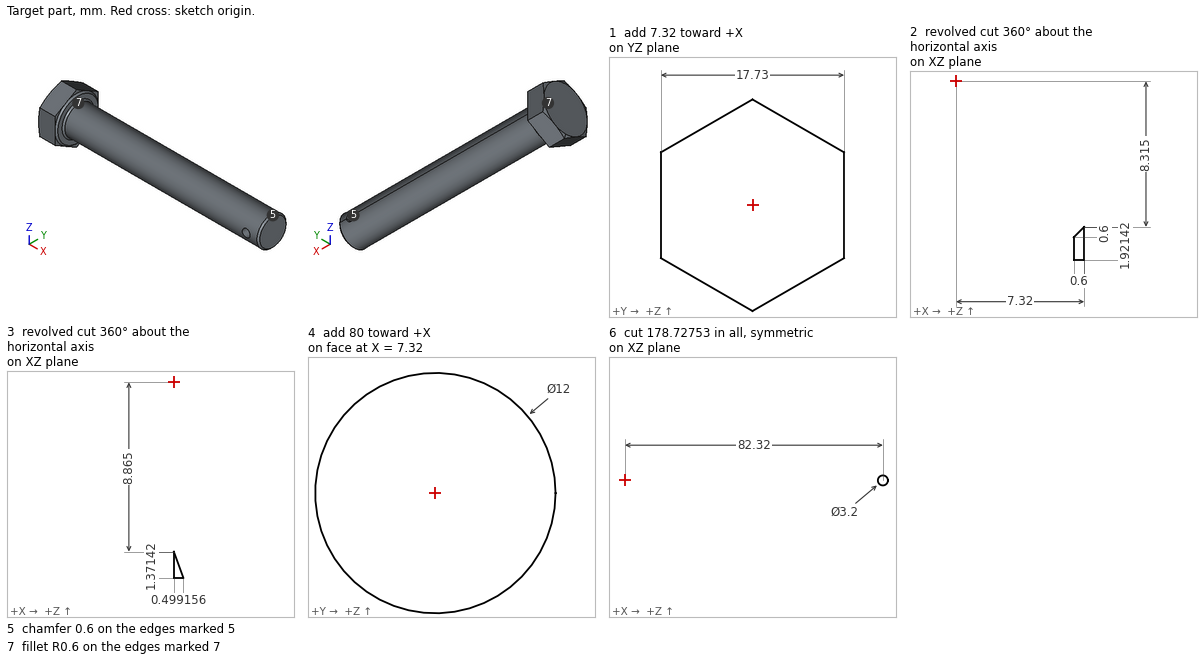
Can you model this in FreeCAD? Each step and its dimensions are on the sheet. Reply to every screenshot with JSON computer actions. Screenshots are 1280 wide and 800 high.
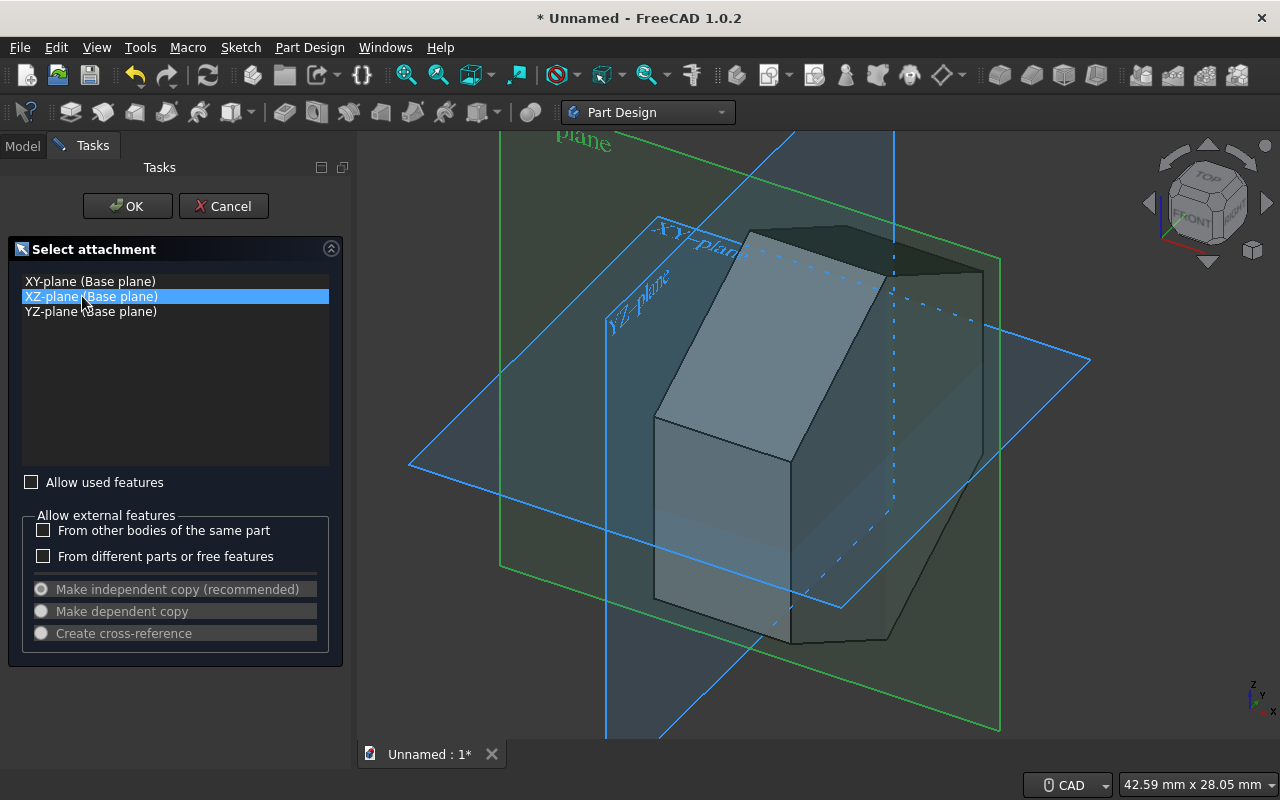
{"action": "left_click", "coordinate": [128, 206]}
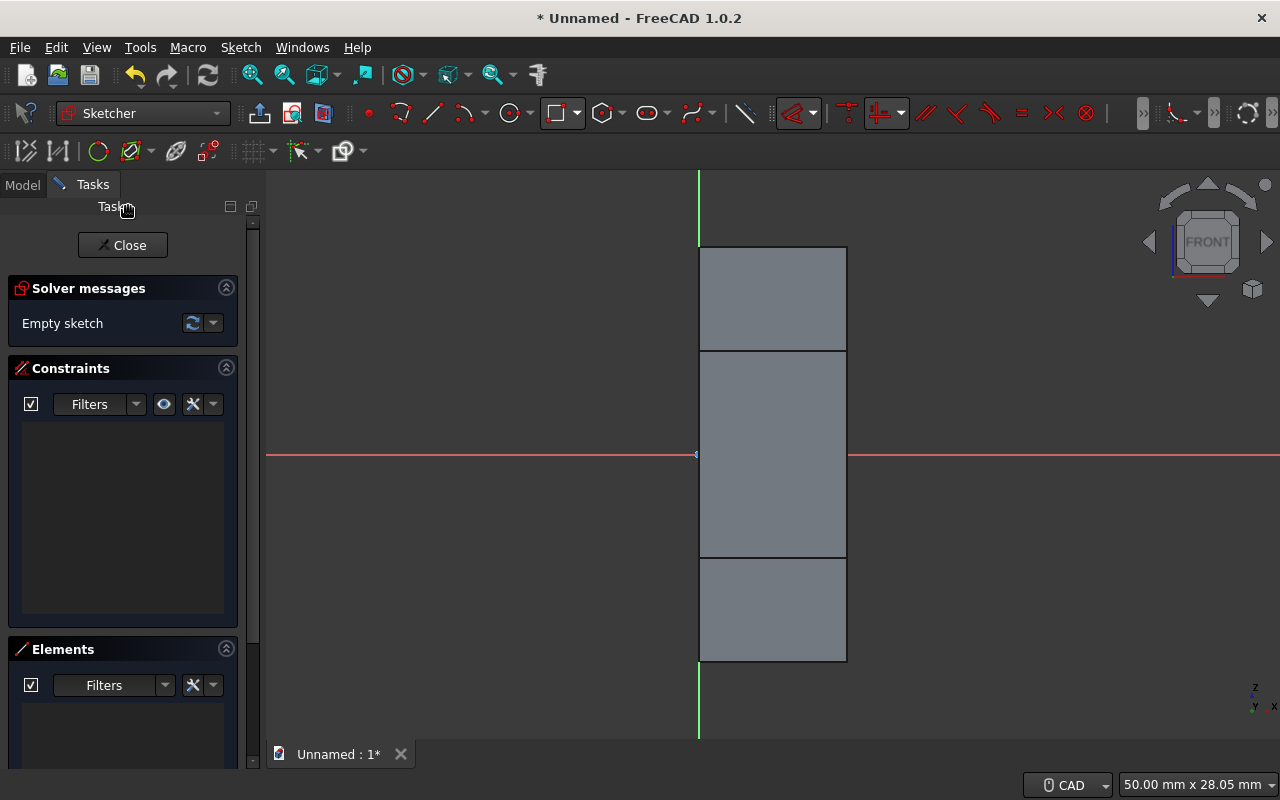
{"action": "left_click", "coordinate": [324, 114]}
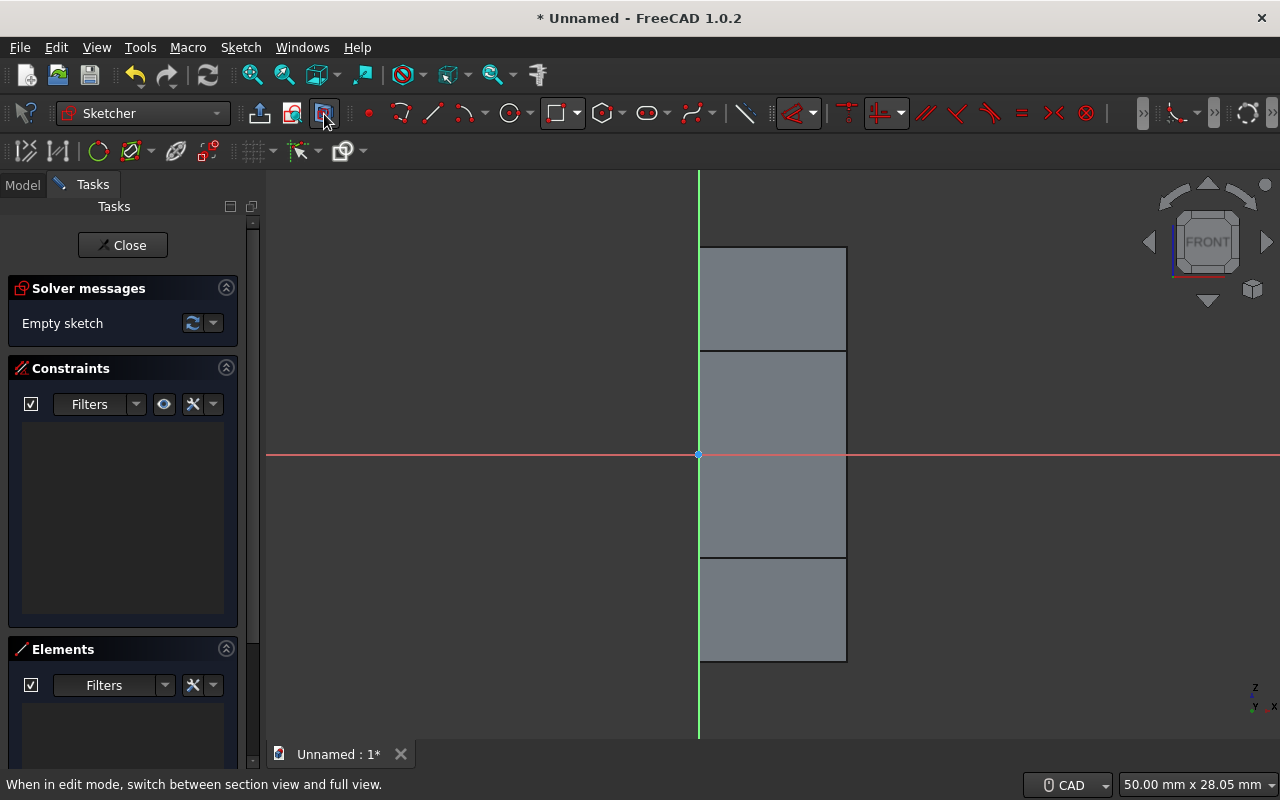
{"action": "scroll", "coordinate": [858, 666], "scroll_direction": "up", "scroll_amount": 11}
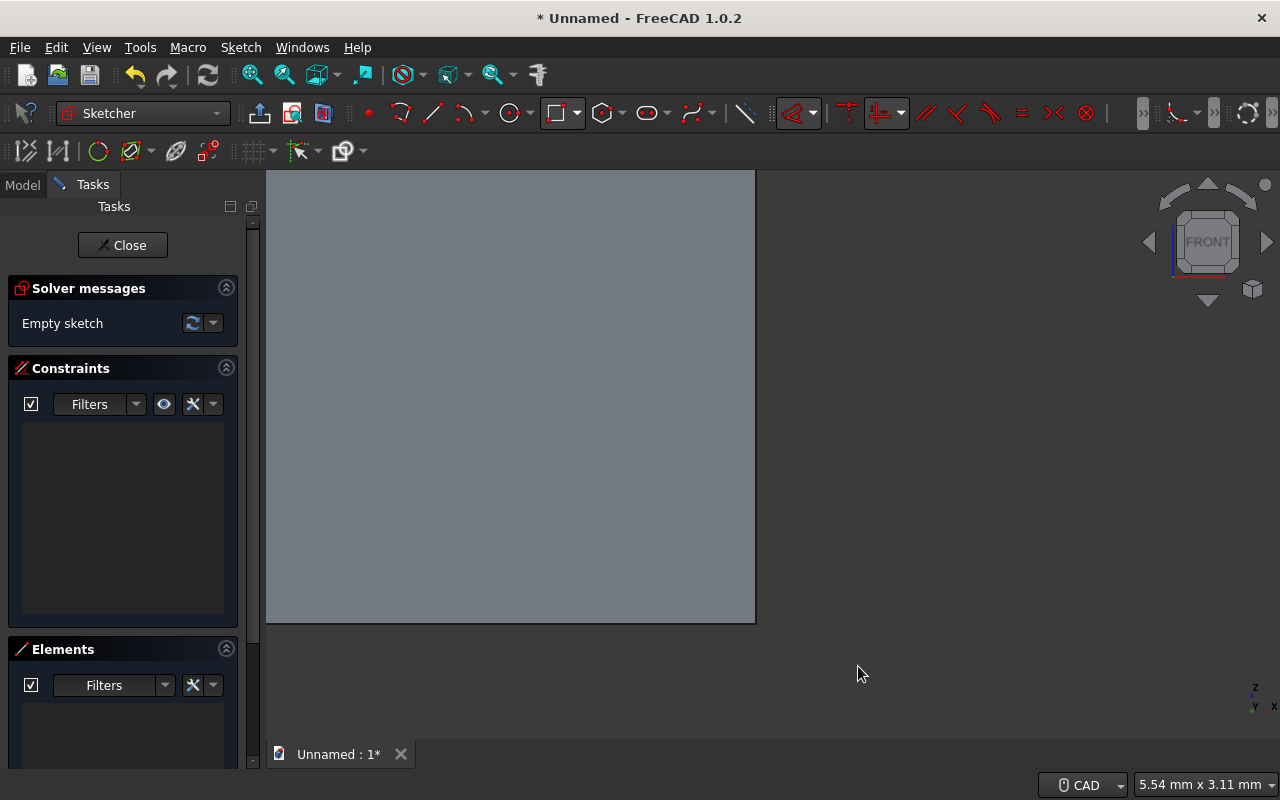
{"action": "left_click", "coordinate": [402, 114]}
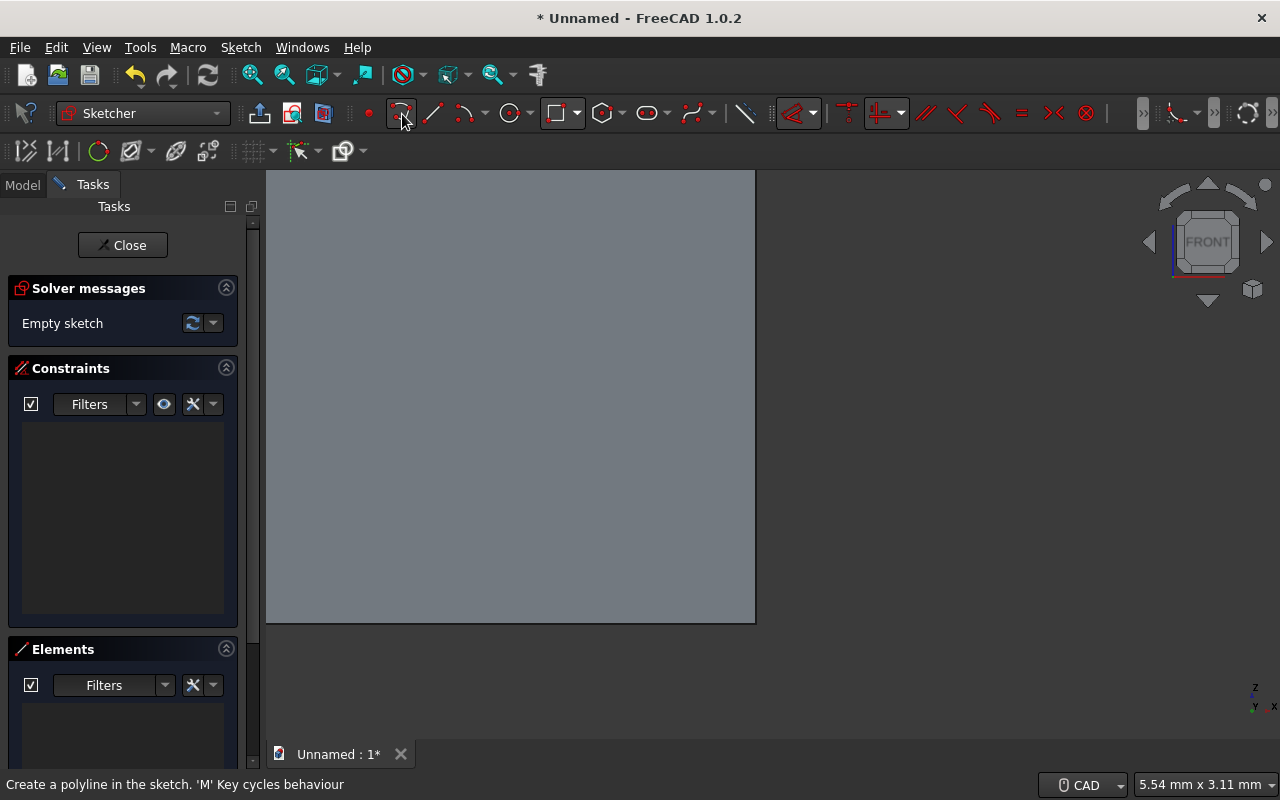
{"action": "left_click", "coordinate": [756, 272]}
{"action": "left_click", "coordinate": [756, 624]}
{"action": "left_click", "coordinate": [646, 624]}
{"action": "left_click", "coordinate": [646, 382]}
{"action": "left_click", "coordinate": [756, 273]}
{"action": "key", "text": "Escape"}
{"action": "key", "text": "Escape"}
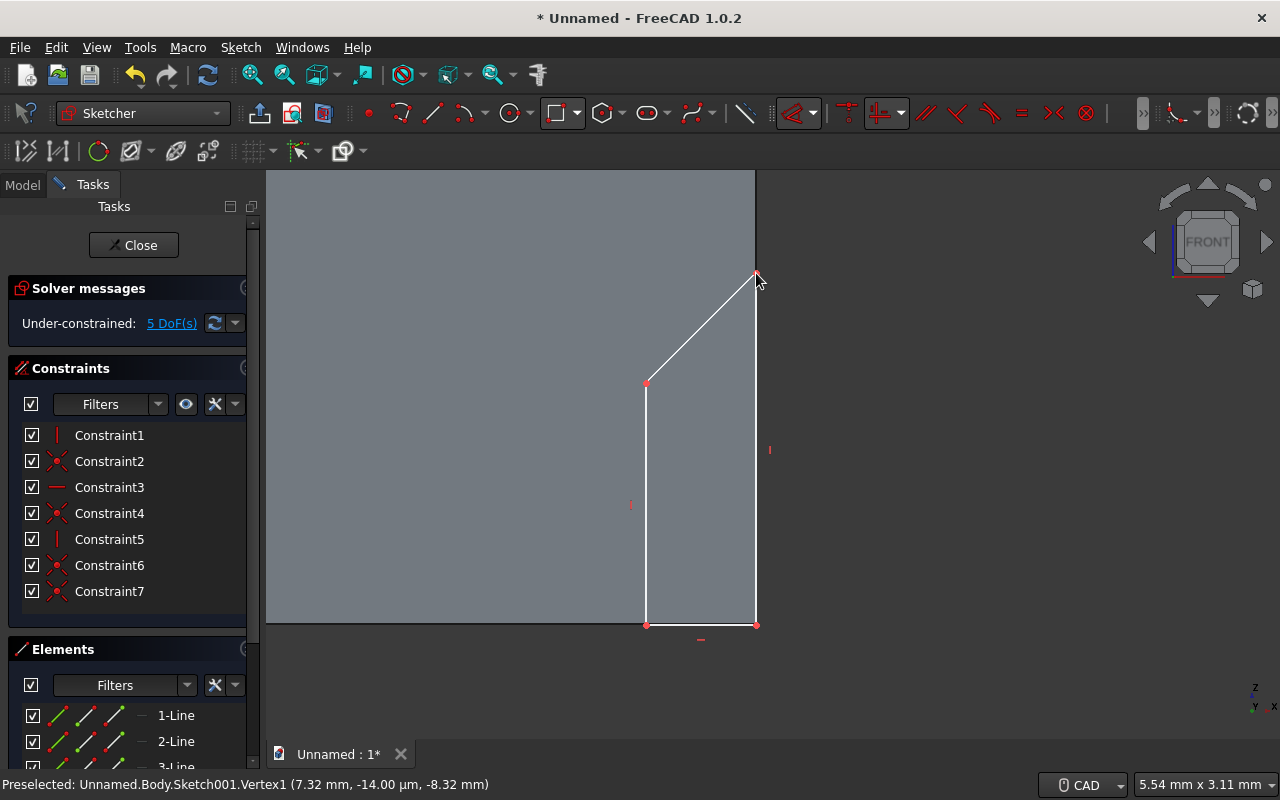
{"action": "left_click", "coordinate": [723, 625]}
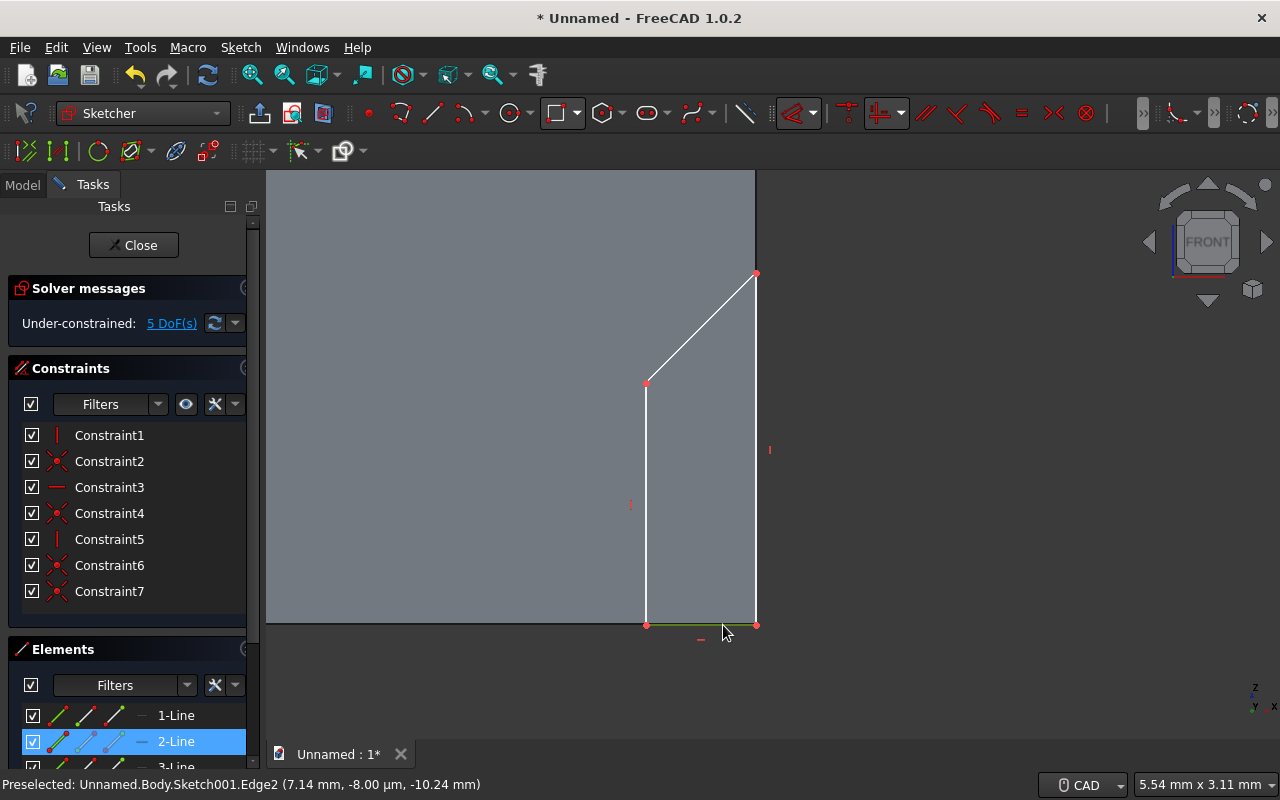
{"action": "left_click", "coordinate": [816, 114]}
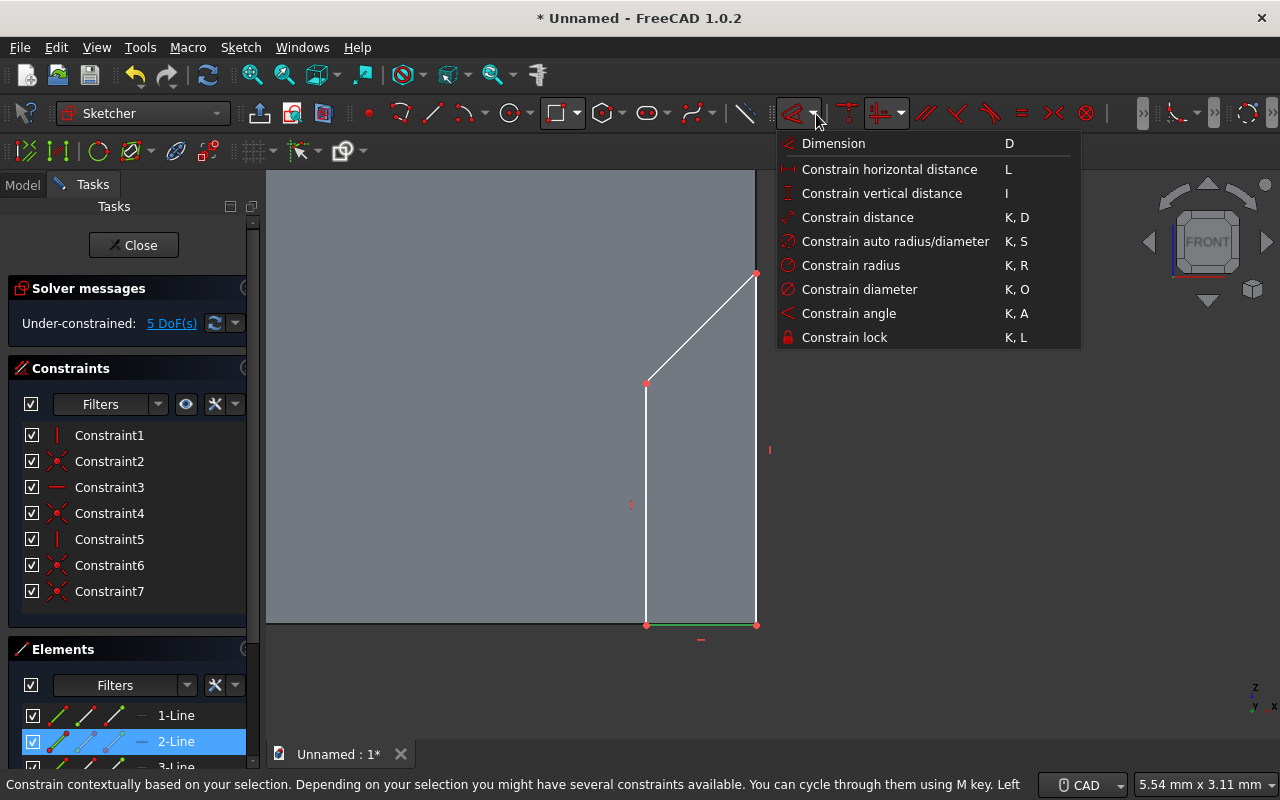
{"action": "left_click", "coordinate": [929, 169]}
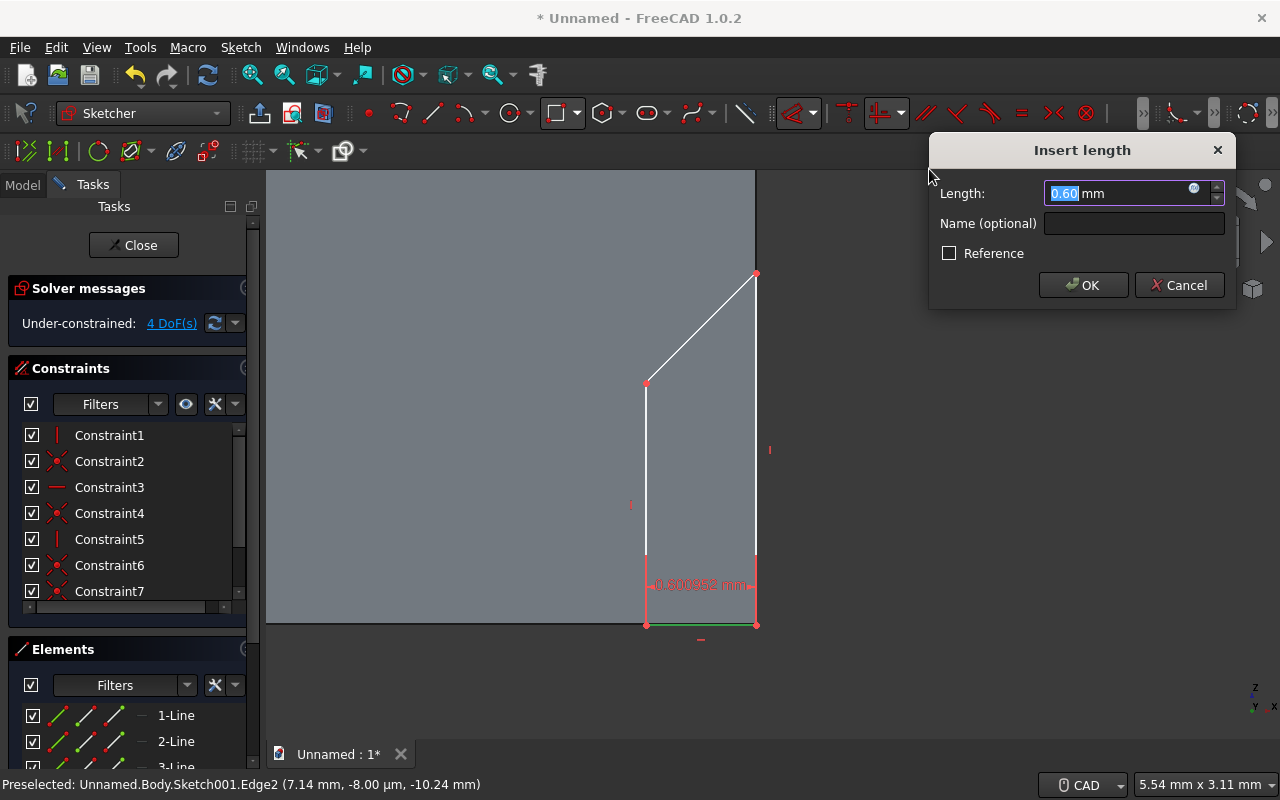
{"action": "type", "text": "0.6"}
{"action": "key", "text": "Return"}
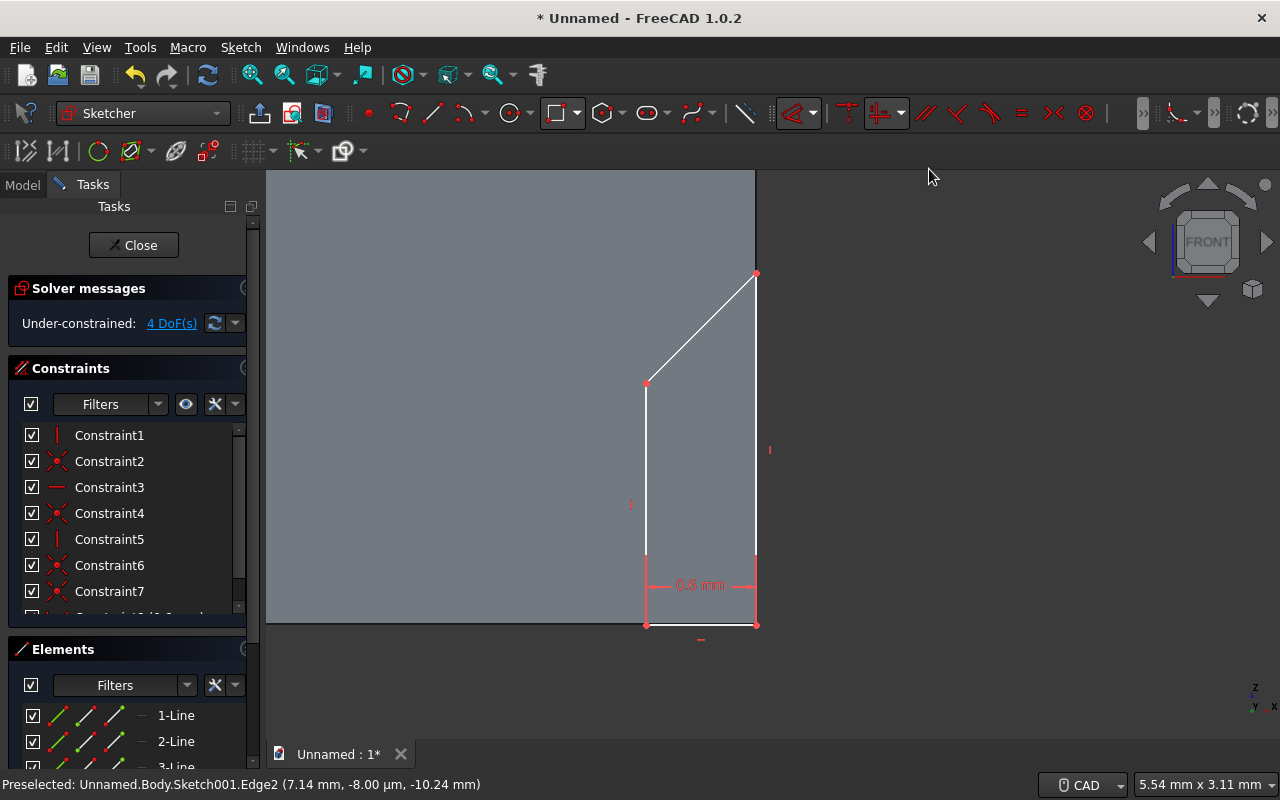
{"action": "left_click", "coordinate": [679, 350]}